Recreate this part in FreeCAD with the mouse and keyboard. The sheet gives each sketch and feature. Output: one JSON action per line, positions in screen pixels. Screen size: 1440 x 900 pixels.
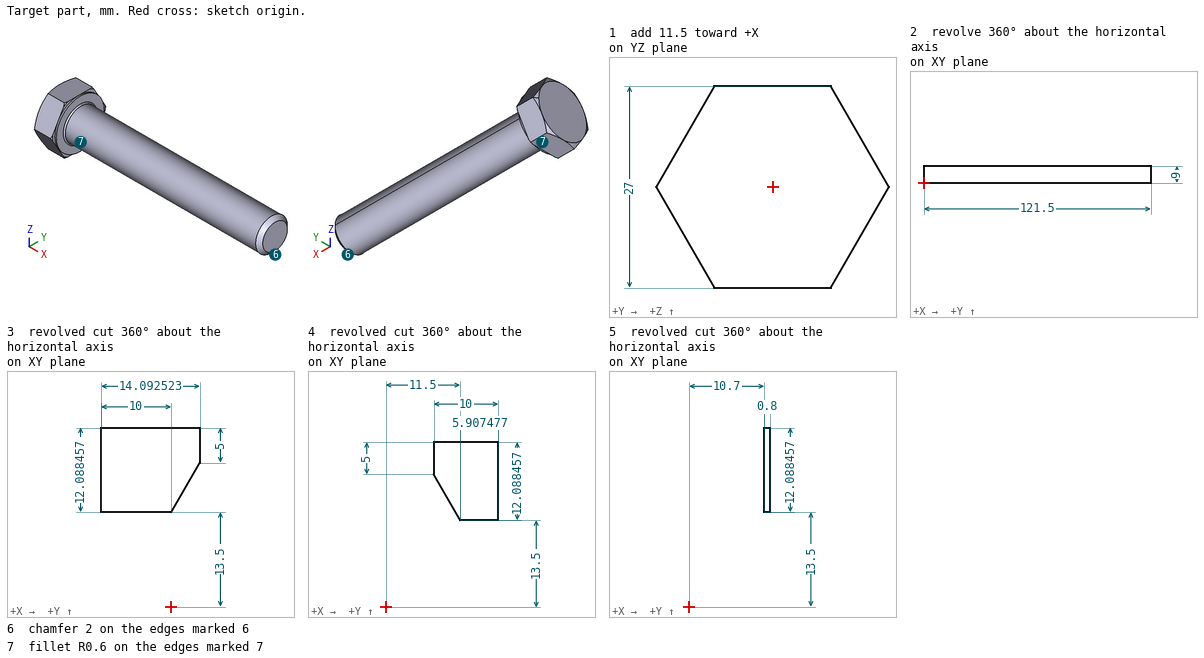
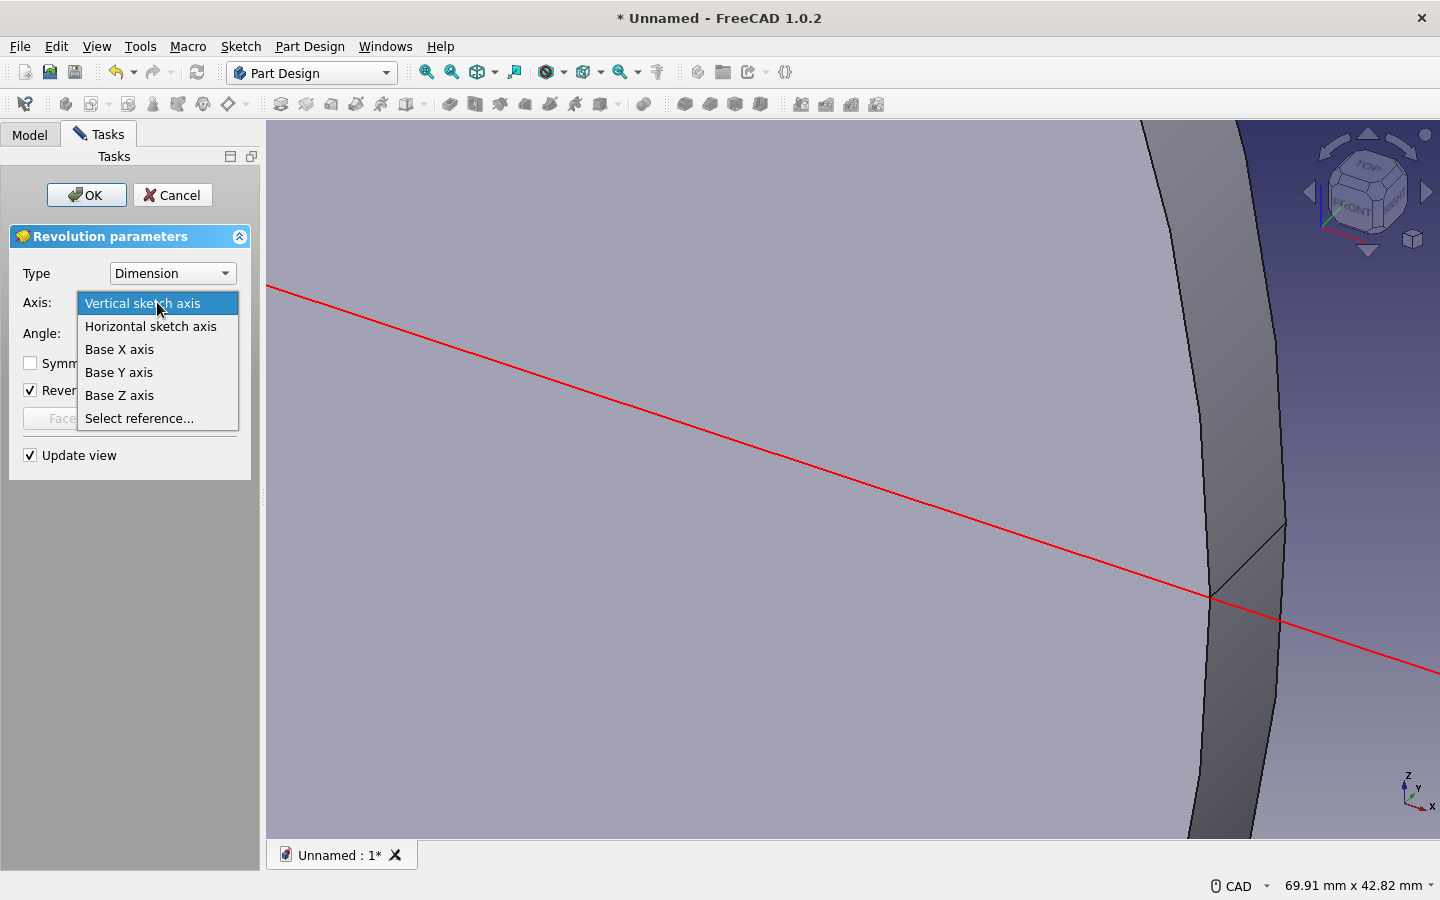
{"action": "left_click", "coordinate": [156, 326]}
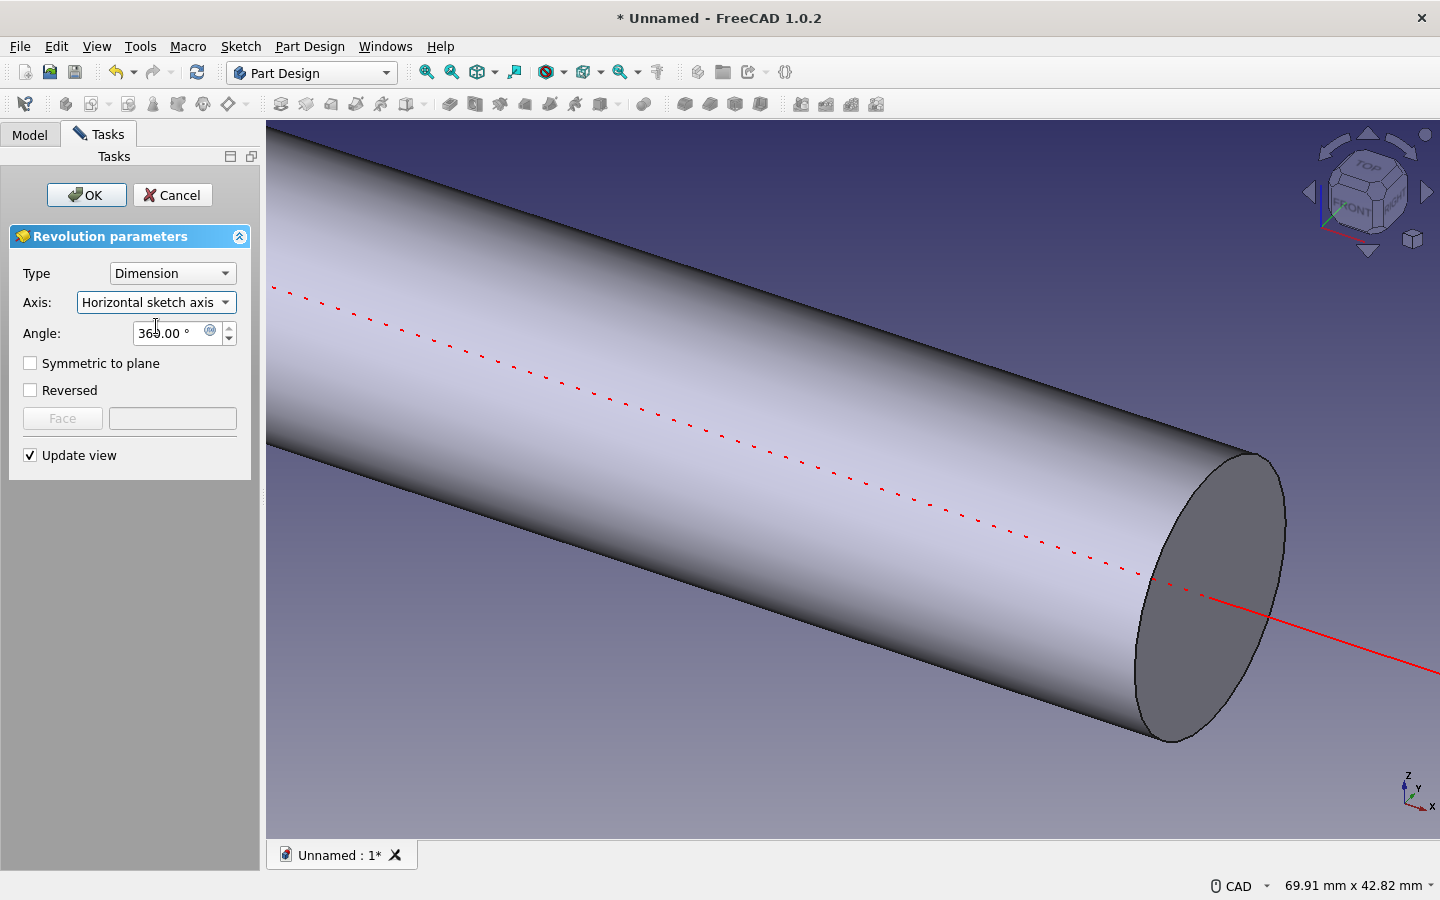
{"action": "left_click", "coordinate": [87, 195]}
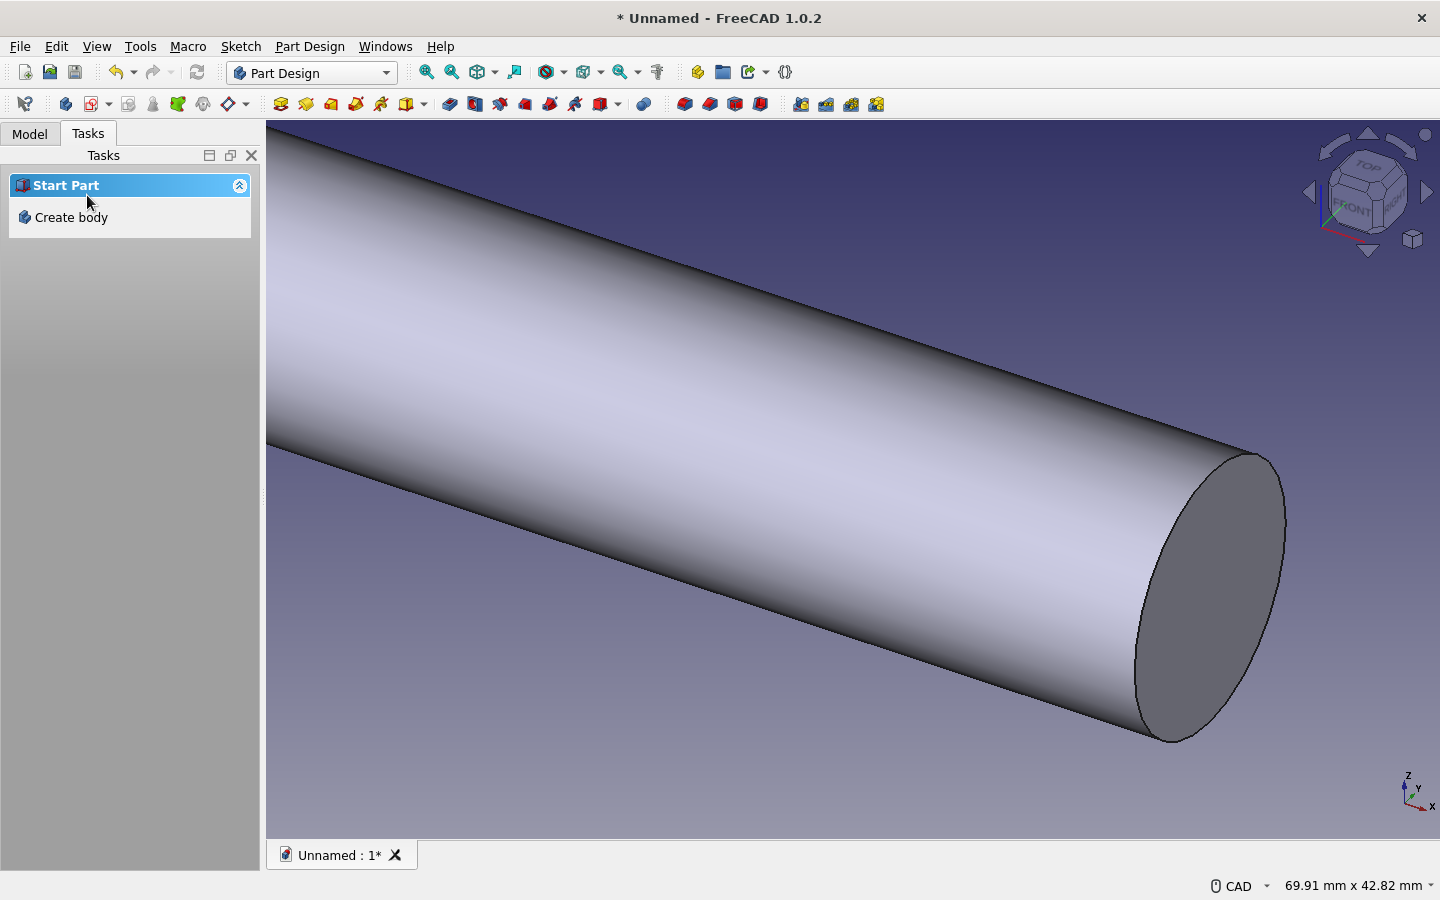
{"action": "left_click", "coordinate": [427, 72]}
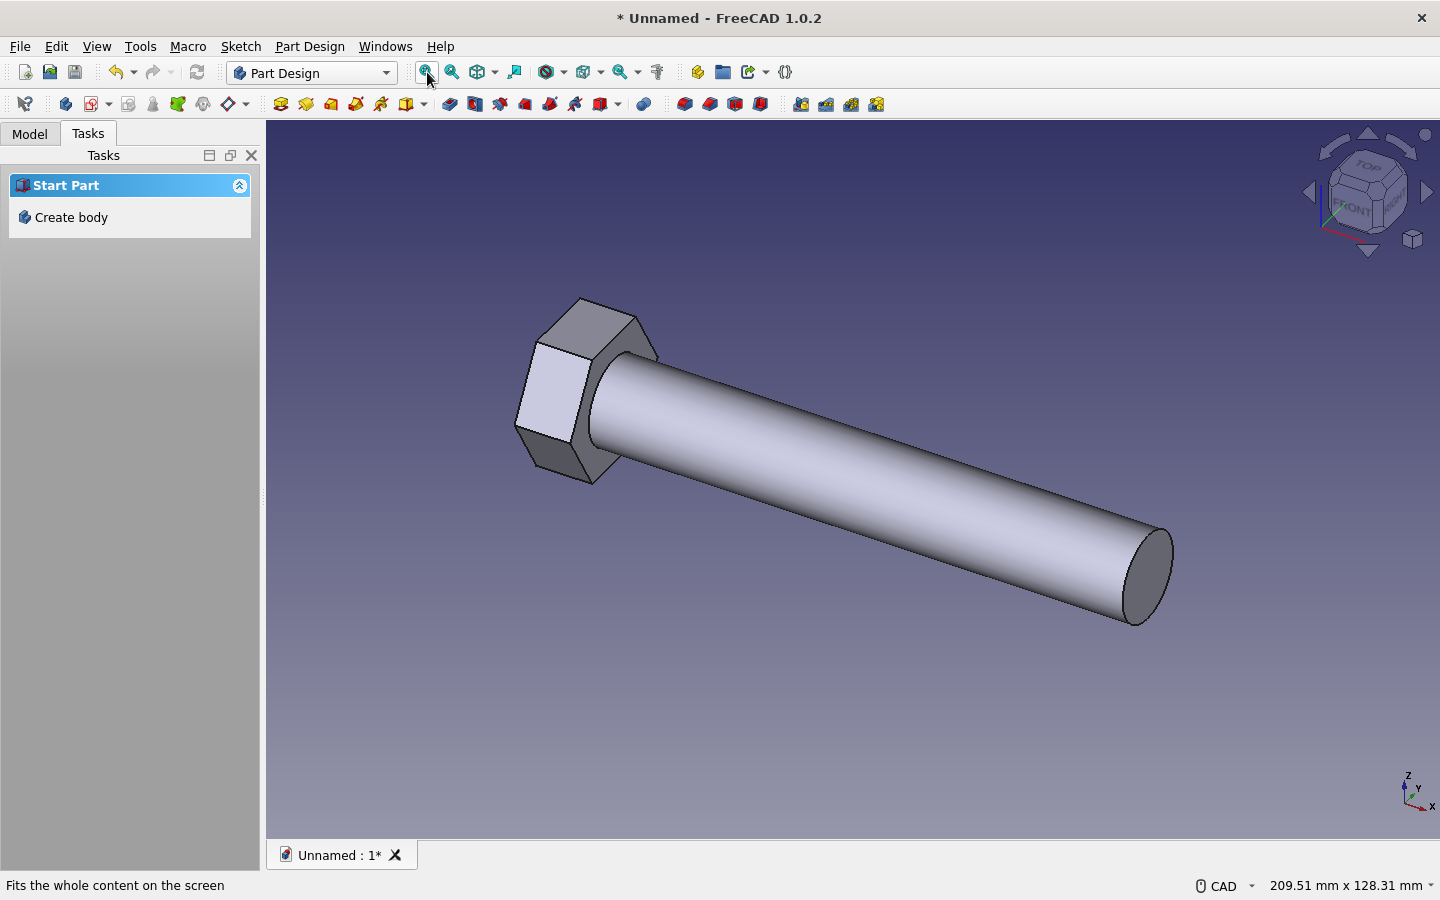
{"action": "left_click", "coordinate": [90, 104]}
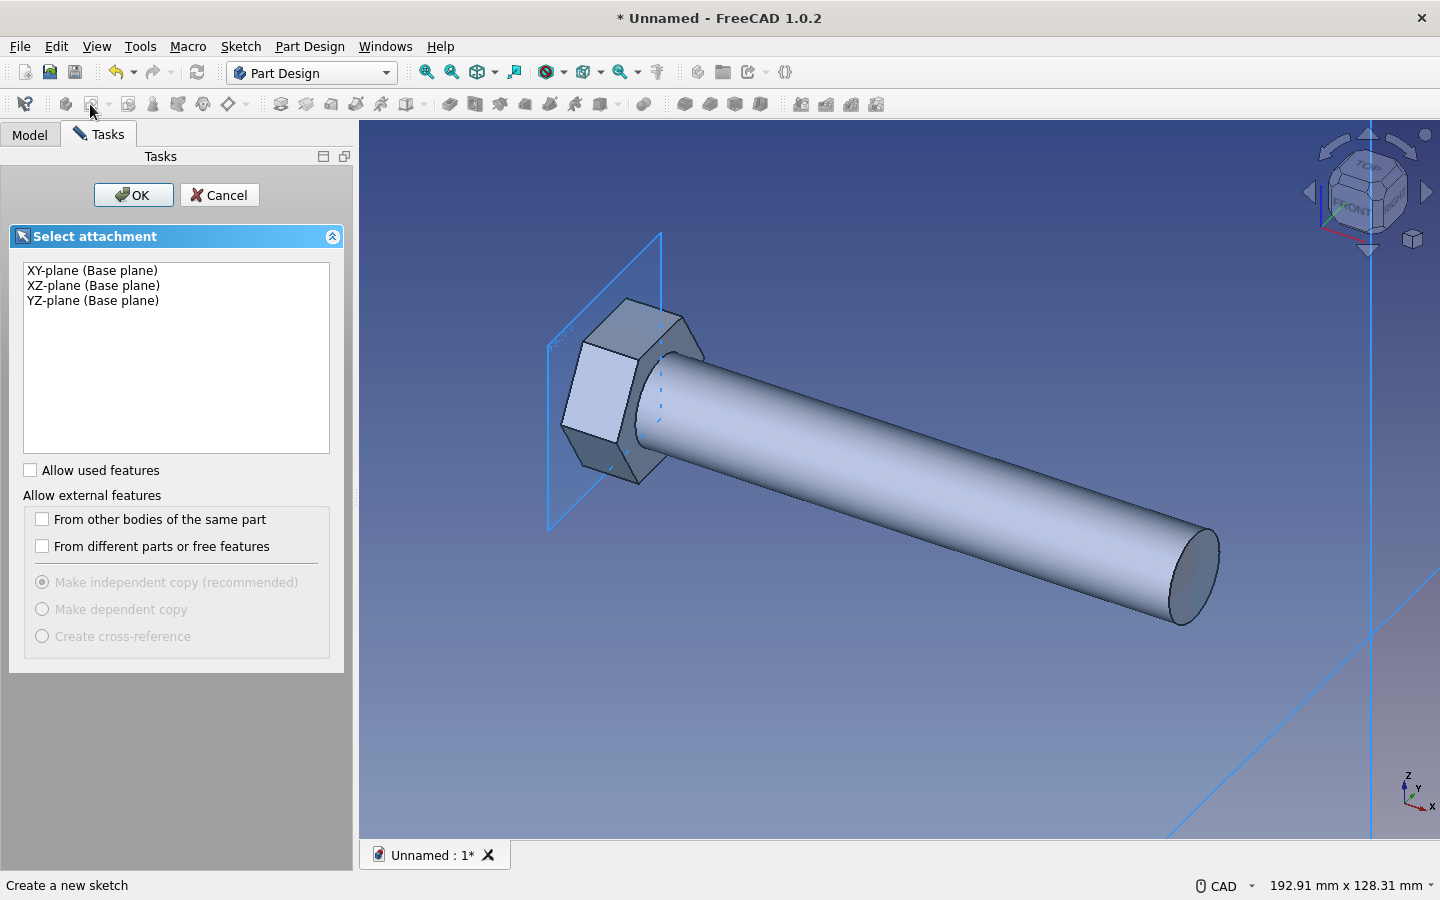
{"action": "left_click", "coordinate": [84, 270]}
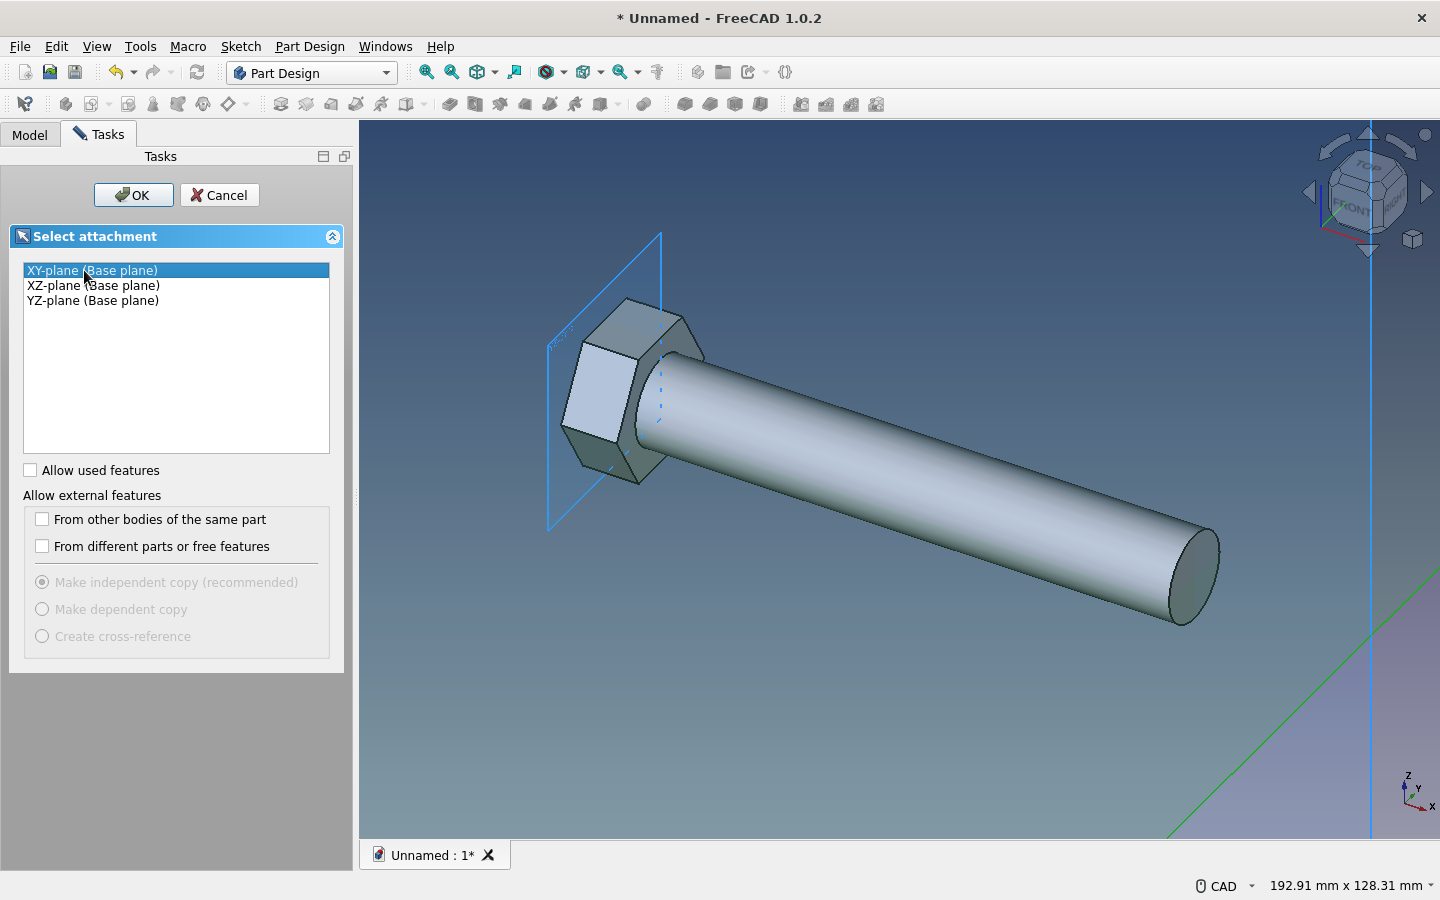
{"action": "left_click", "coordinate": [134, 195]}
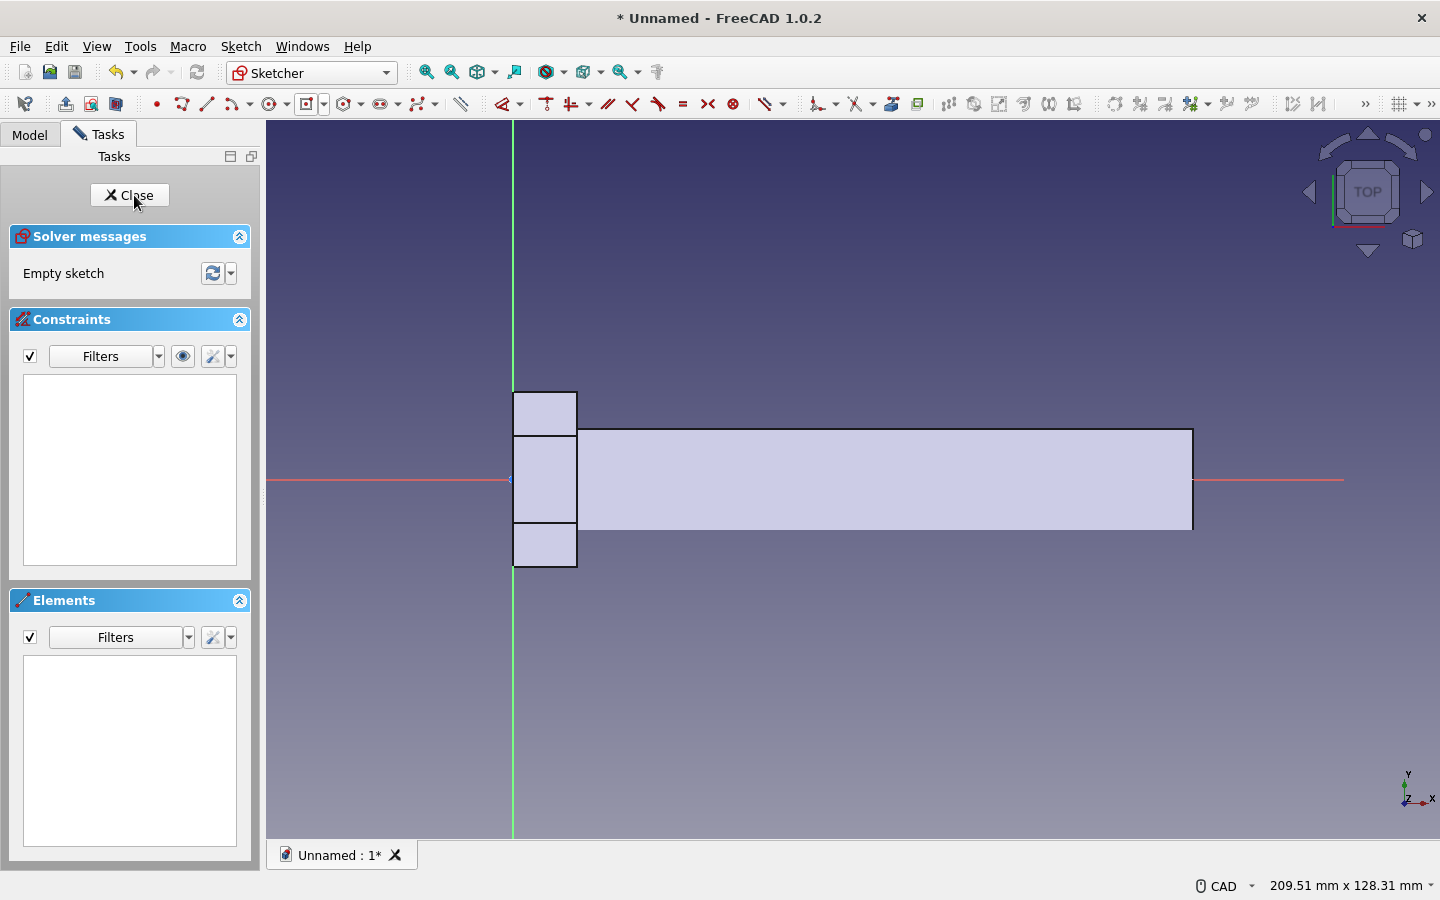
{"action": "left_click", "coordinate": [116, 104]}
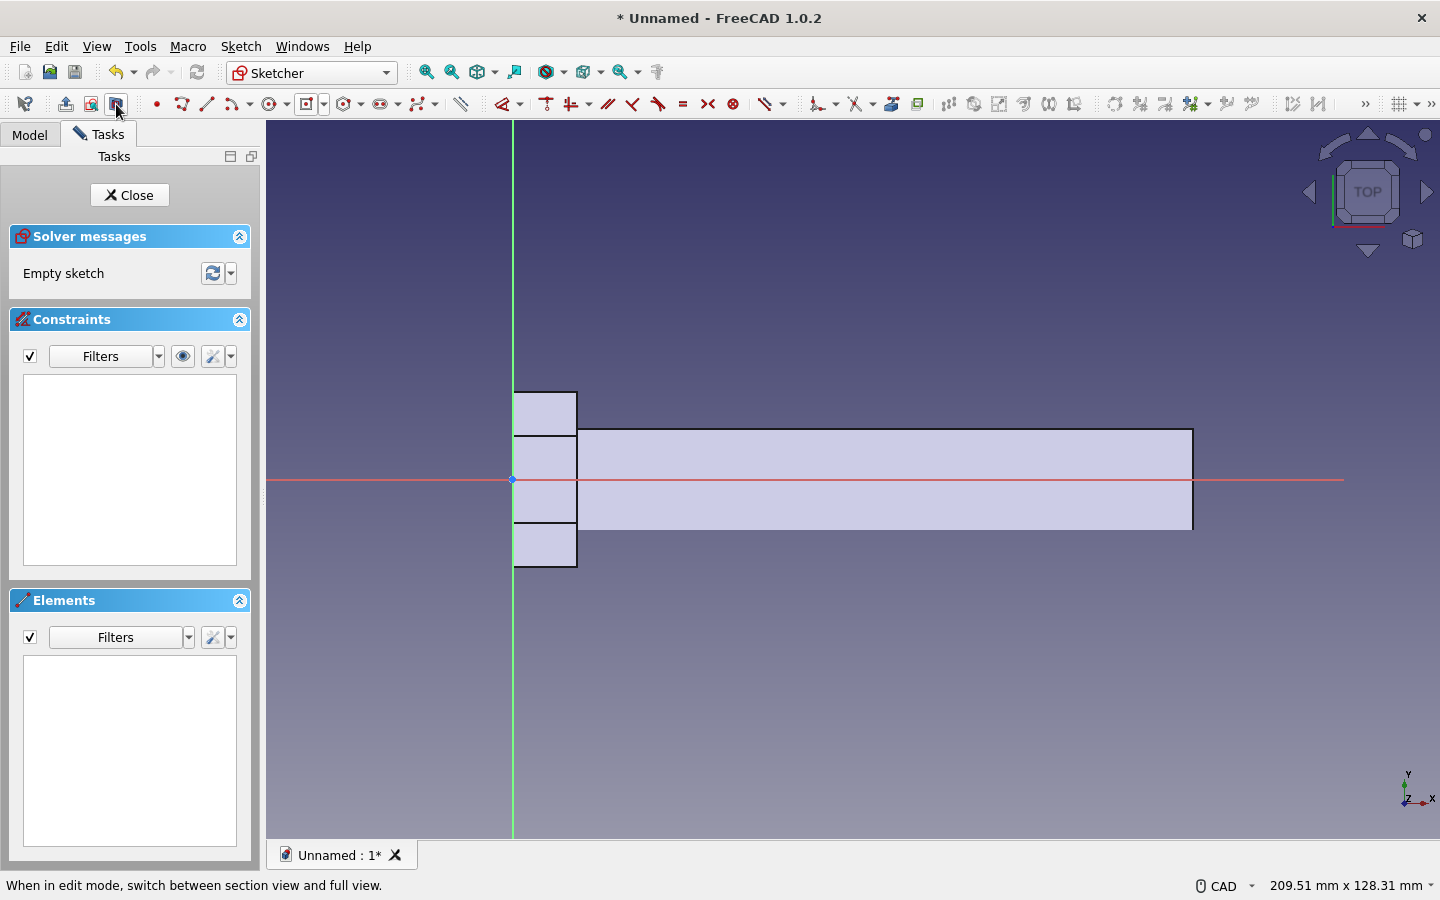
{"action": "scroll", "coordinate": [372, 377], "scroll_direction": "up", "scroll_amount": 6}